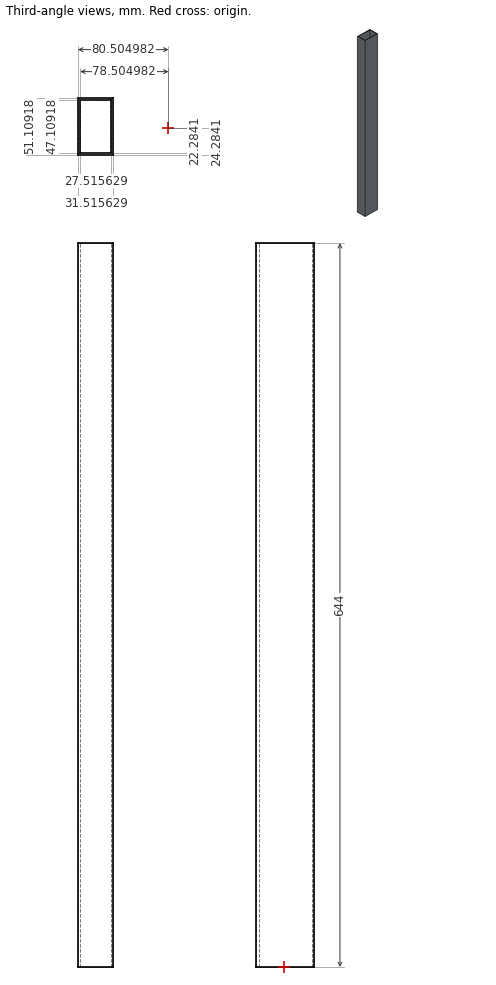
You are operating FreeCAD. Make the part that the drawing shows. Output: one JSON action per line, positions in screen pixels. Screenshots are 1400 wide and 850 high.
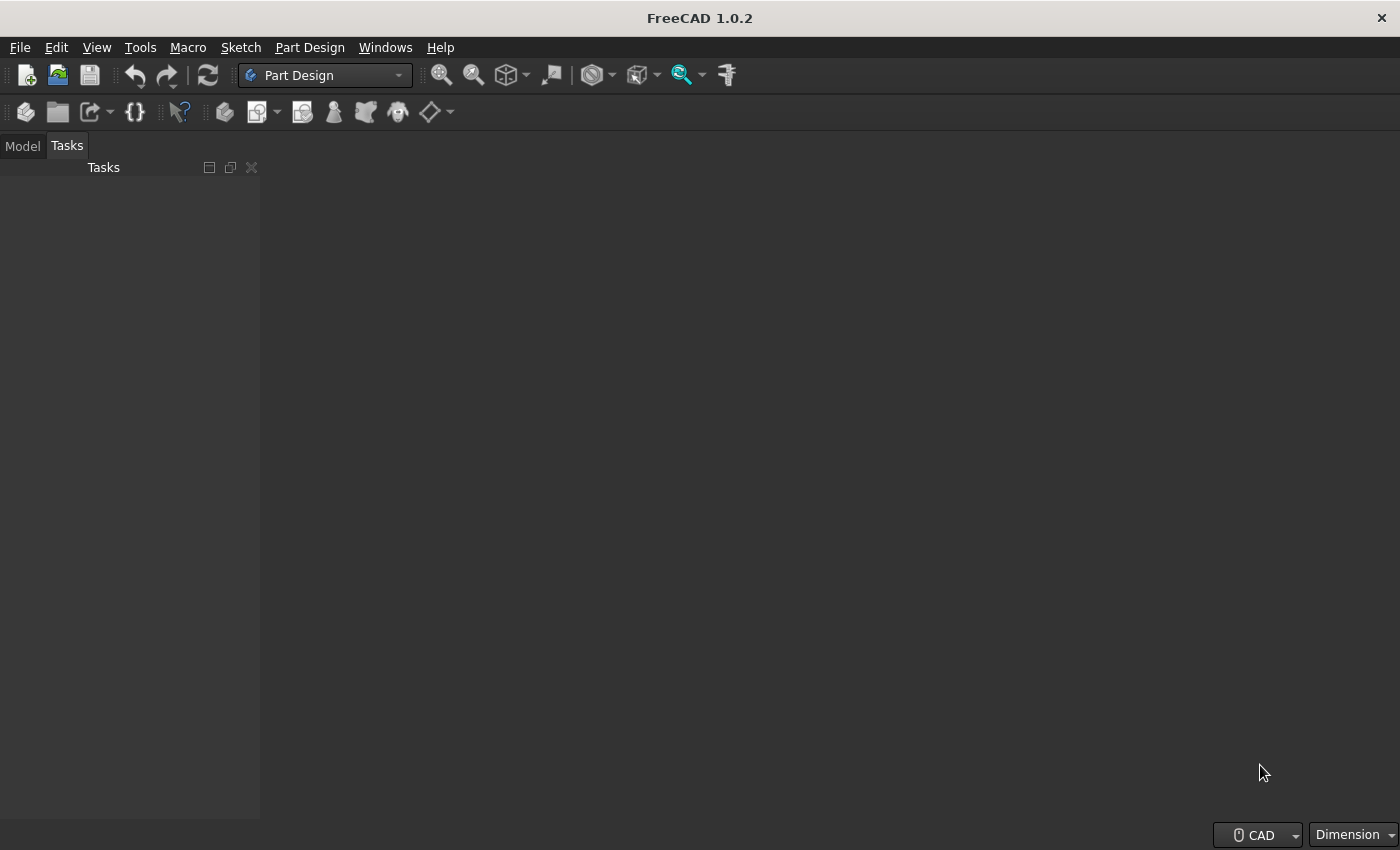
{"action": "key", "text": "ctrl+n"}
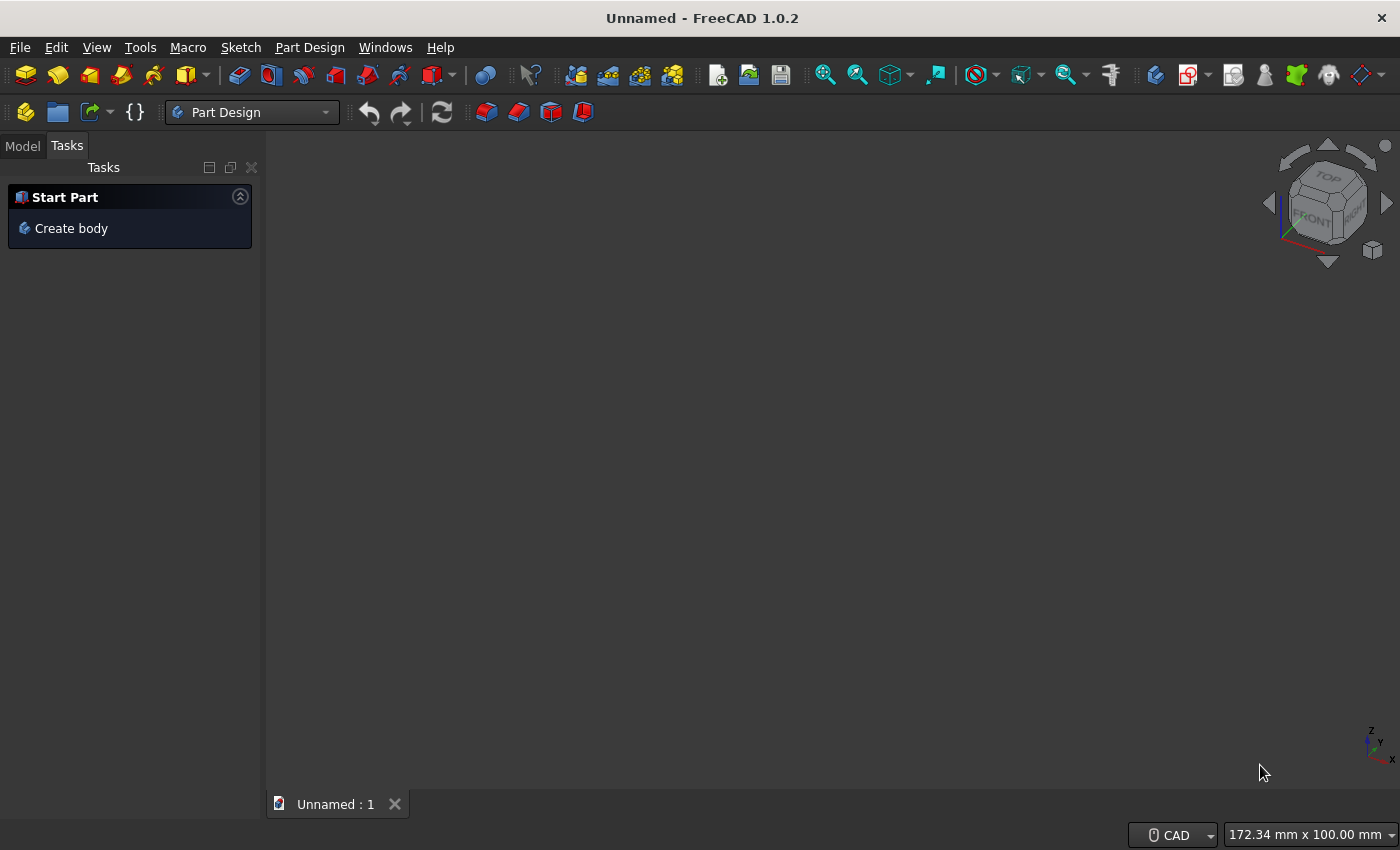
{"action": "left_click", "coordinate": [1188, 76]}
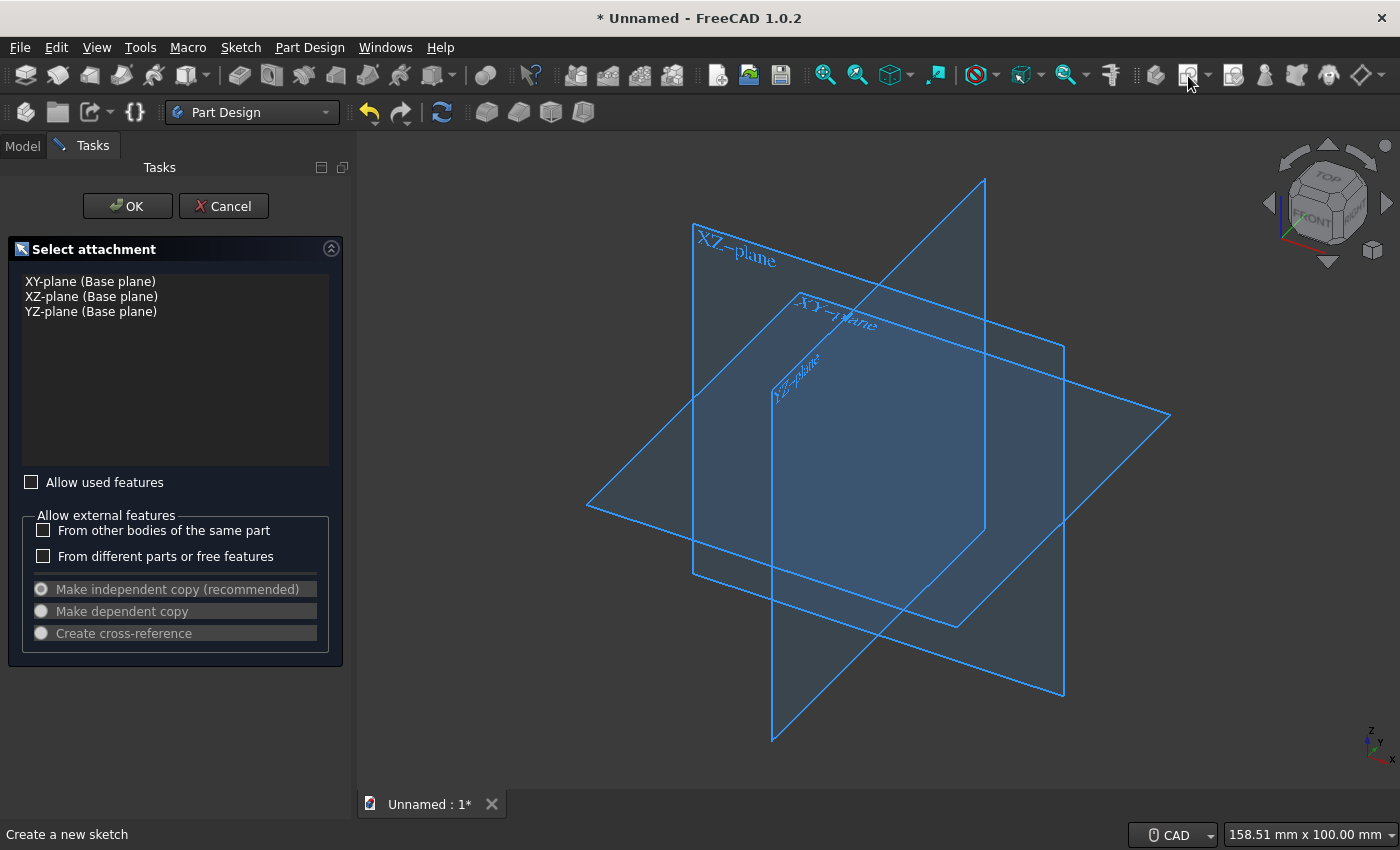
{"action": "left_click", "coordinate": [82, 282]}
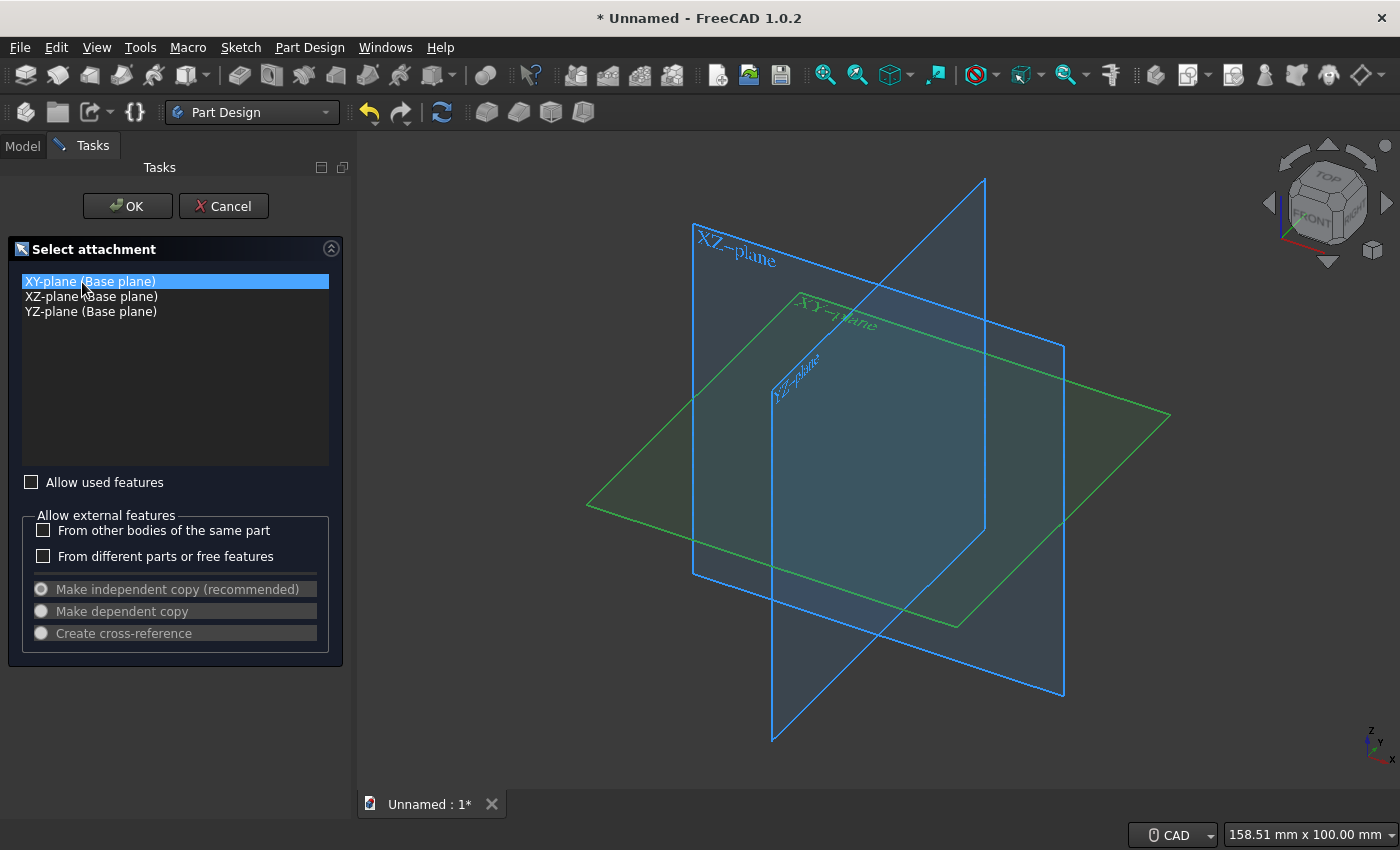
{"action": "left_click", "coordinate": [128, 206]}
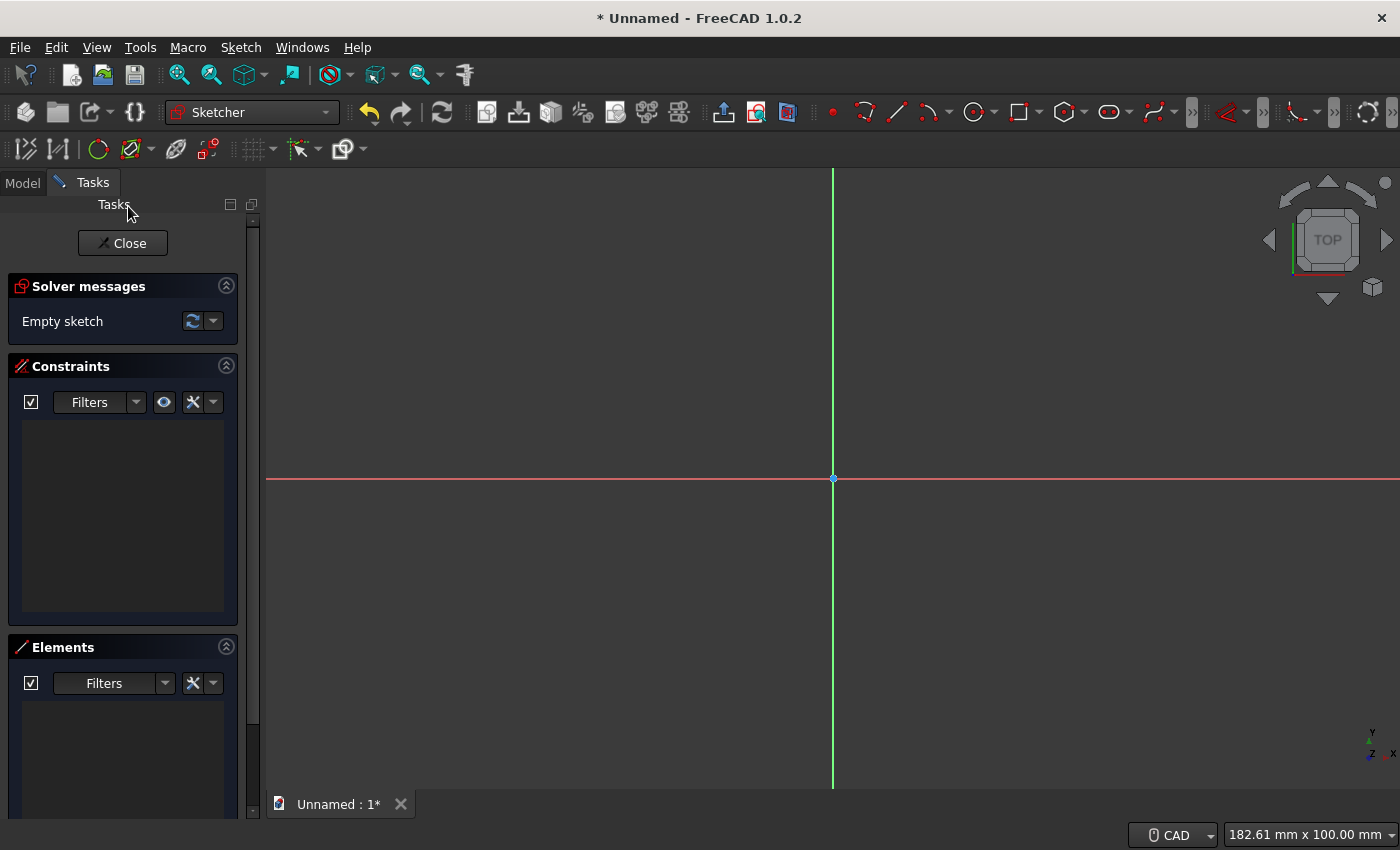
{"action": "left_click", "coordinate": [1020, 112]}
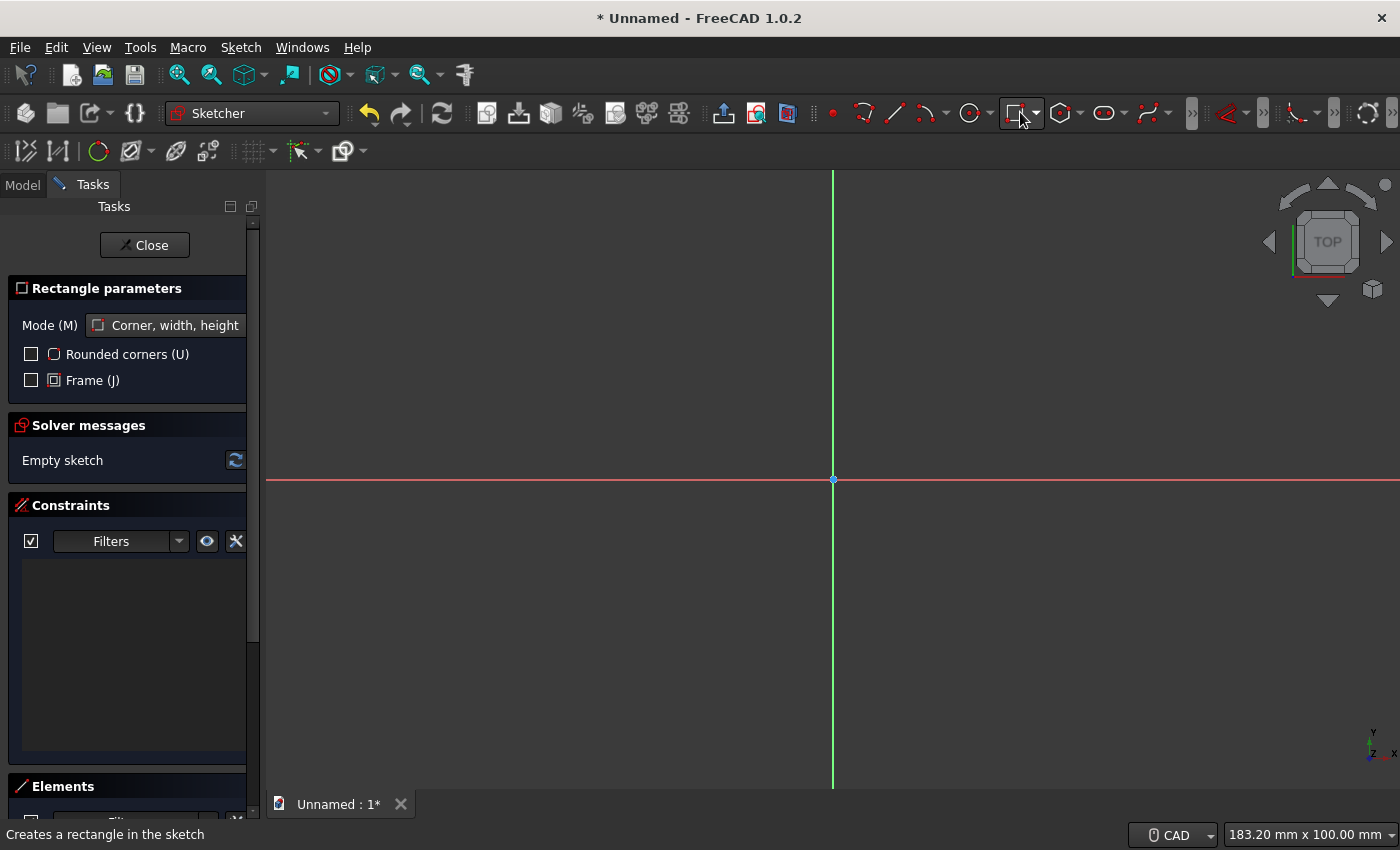
{"action": "left_click", "coordinate": [335, 313]}
{"action": "mouse_move", "coordinate": [530, 630]}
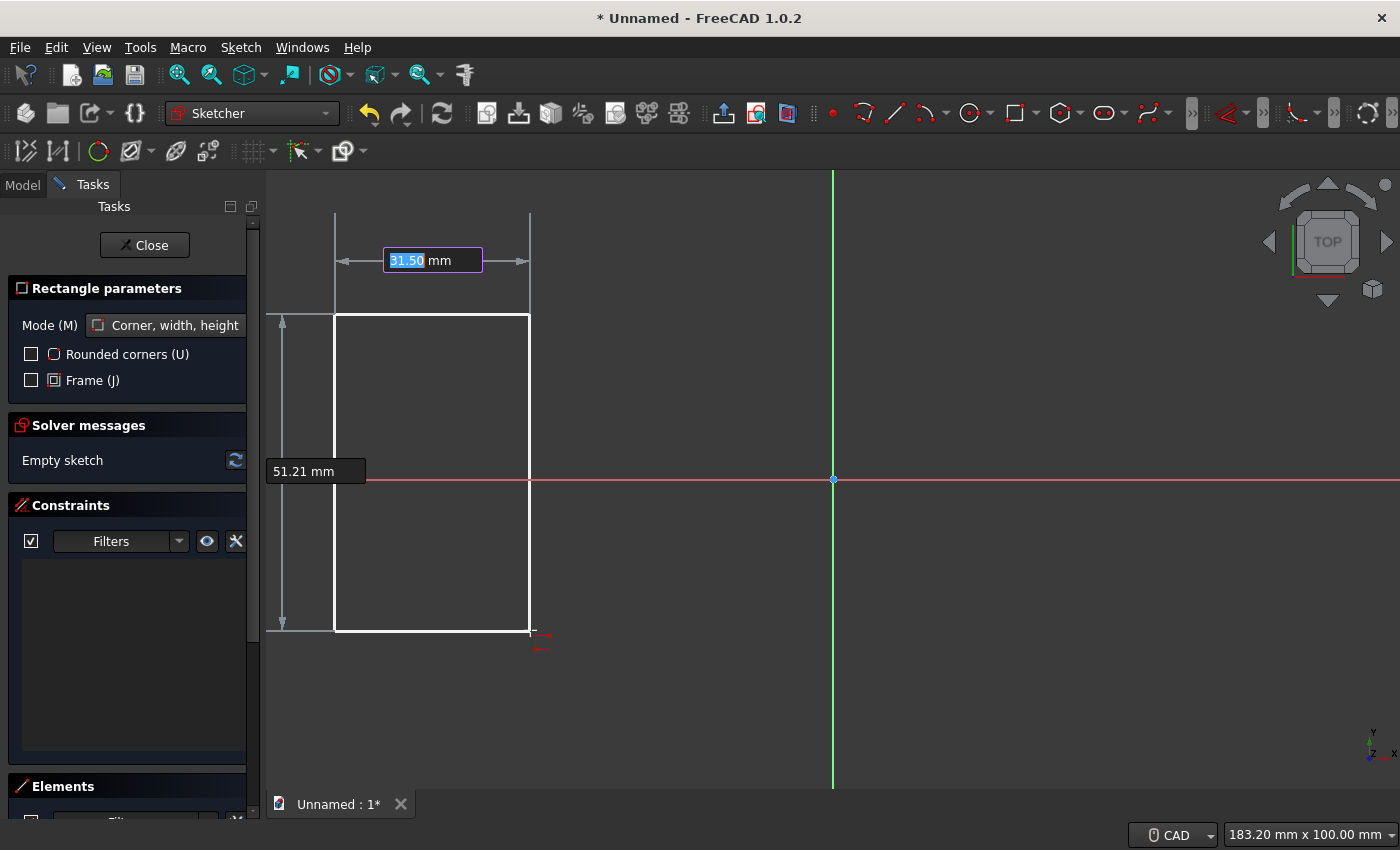
{"action": "type", "text": "31.515629"}
{"action": "key", "text": "Tab"}
{"action": "type", "text": "51.10918"}
{"action": "key", "text": "Return"}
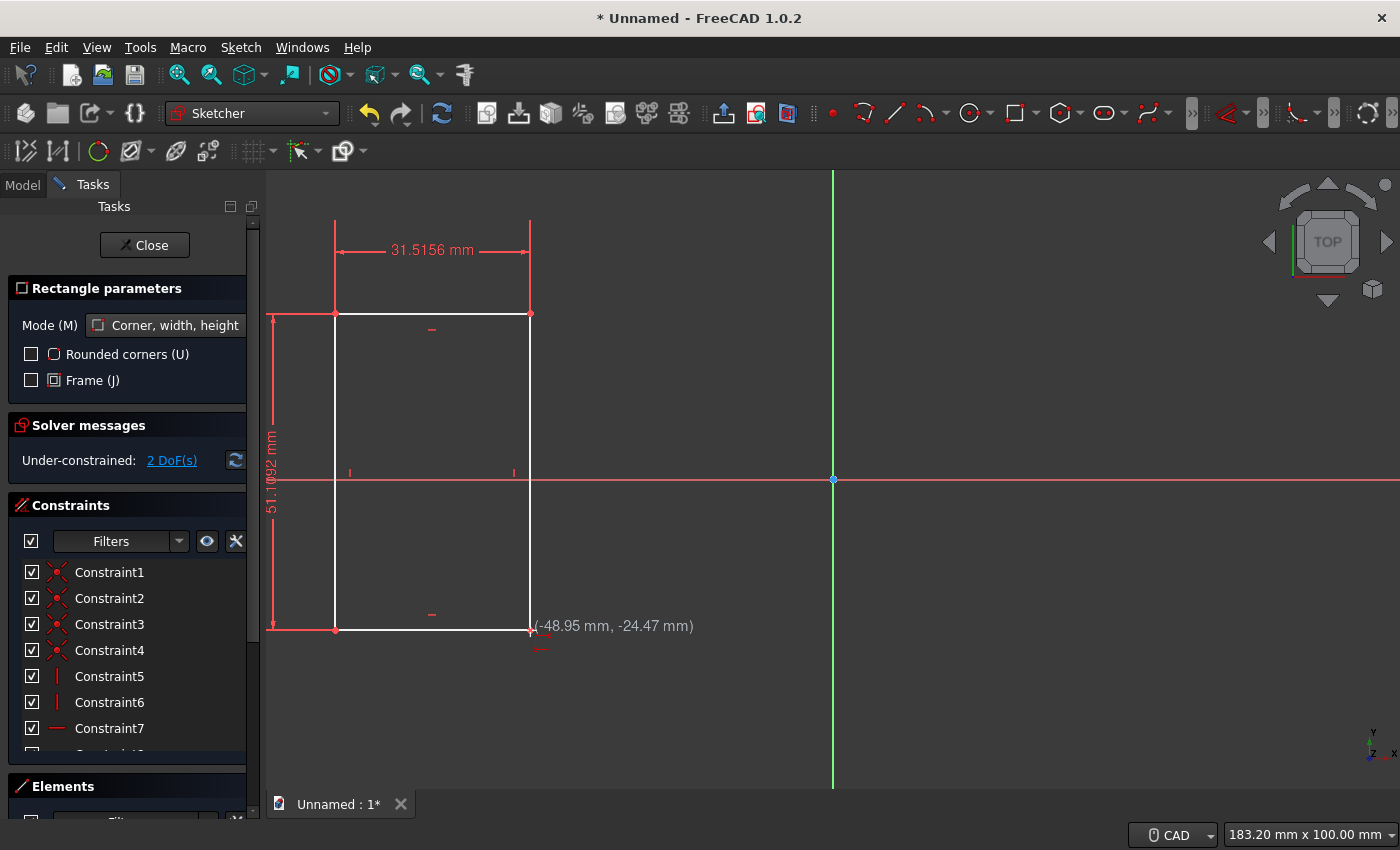
{"action": "scroll", "coordinate": [347, 326], "scroll_direction": "up", "scroll_amount": 2}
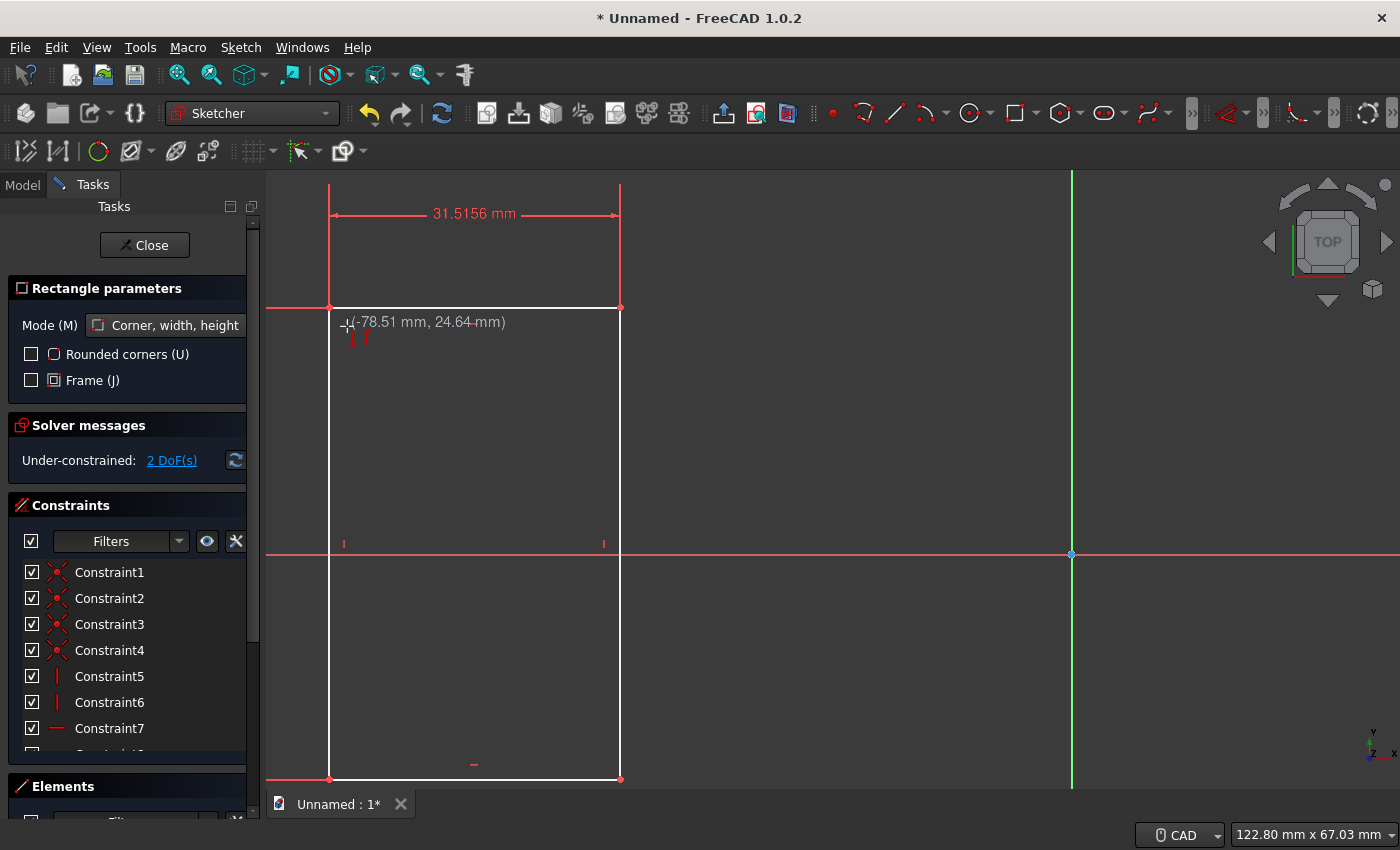
{"action": "left_click", "coordinate": [347, 326]}
{"action": "mouse_move", "coordinate": [601, 761]}